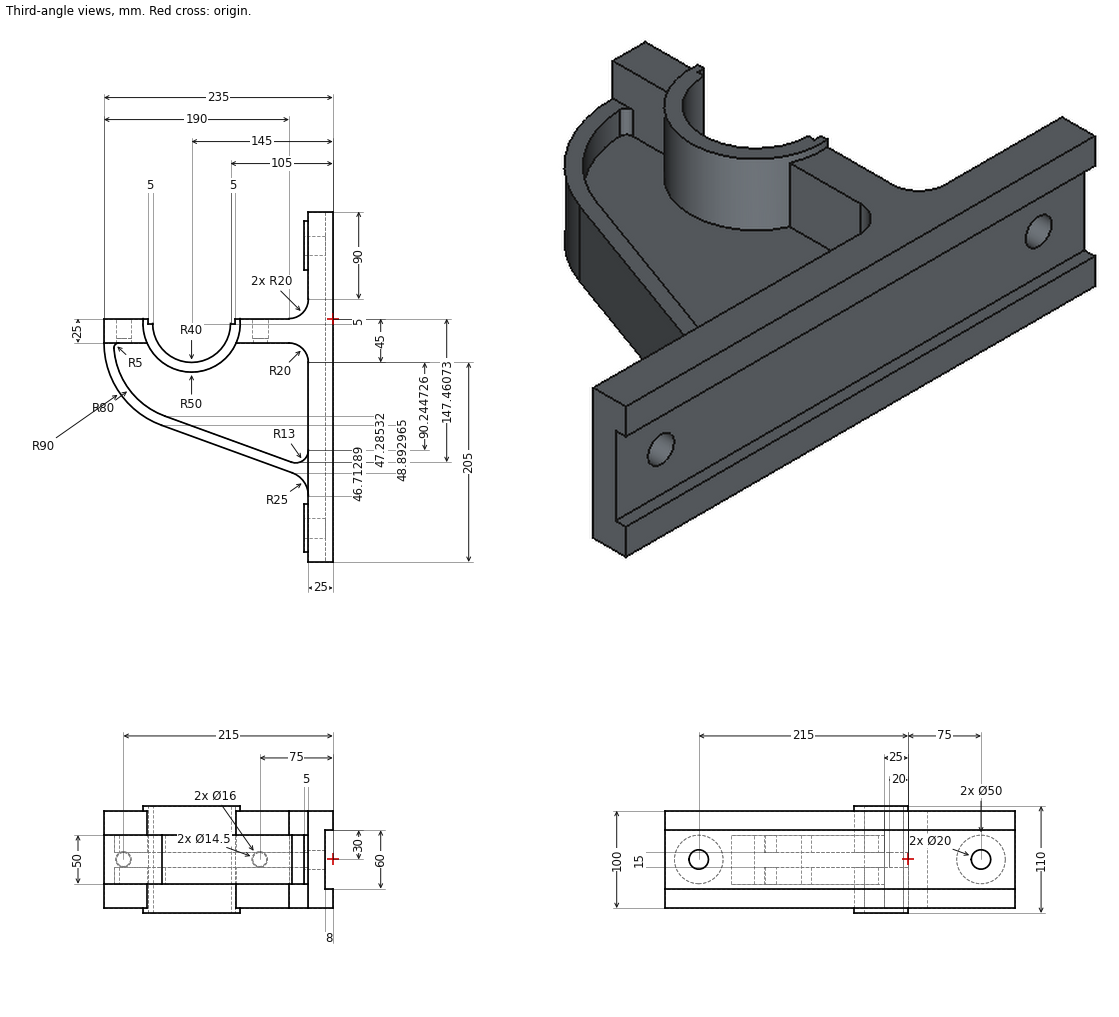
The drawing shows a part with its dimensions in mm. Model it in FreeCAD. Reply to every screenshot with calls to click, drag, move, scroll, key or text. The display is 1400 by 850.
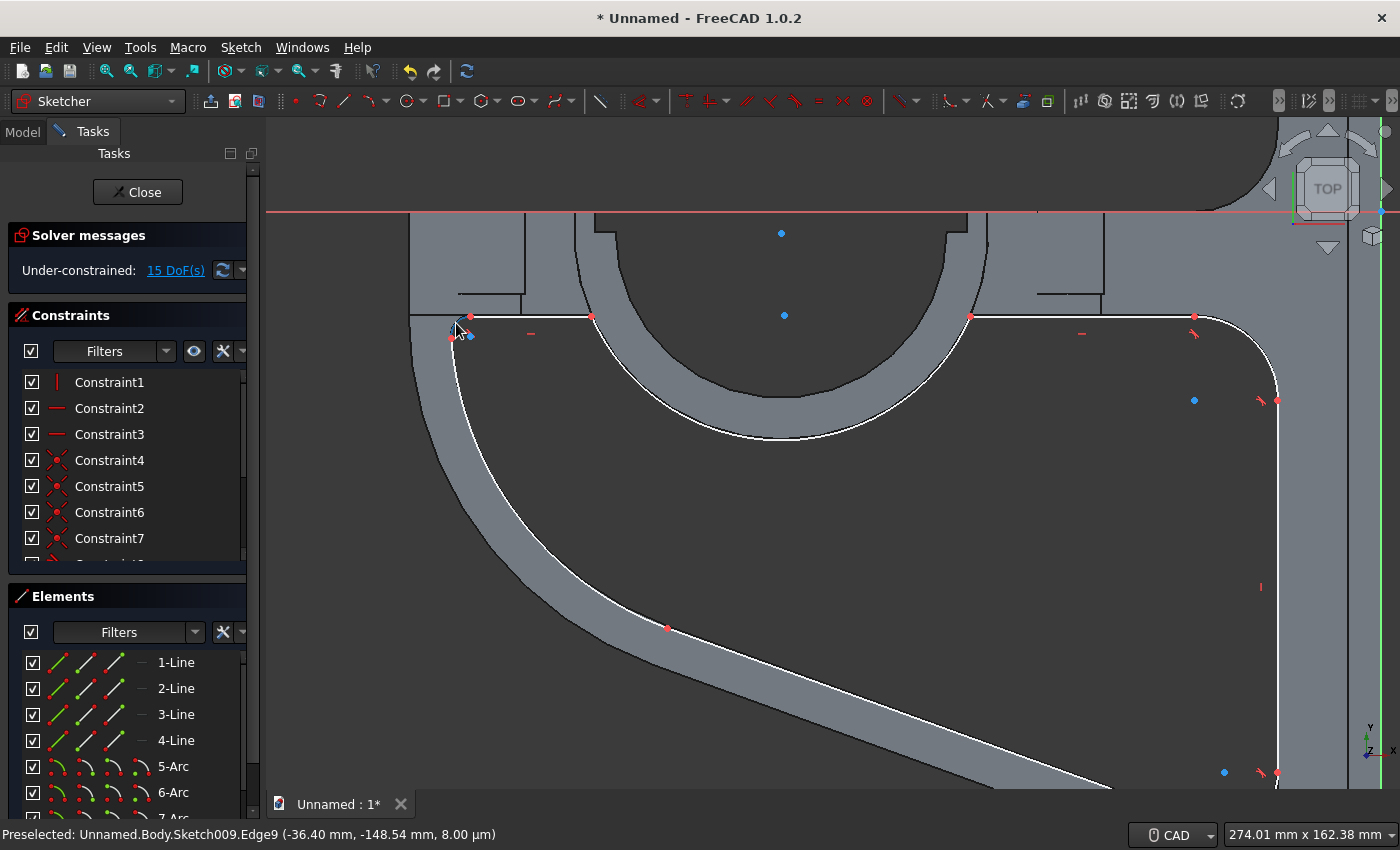
click(456, 323)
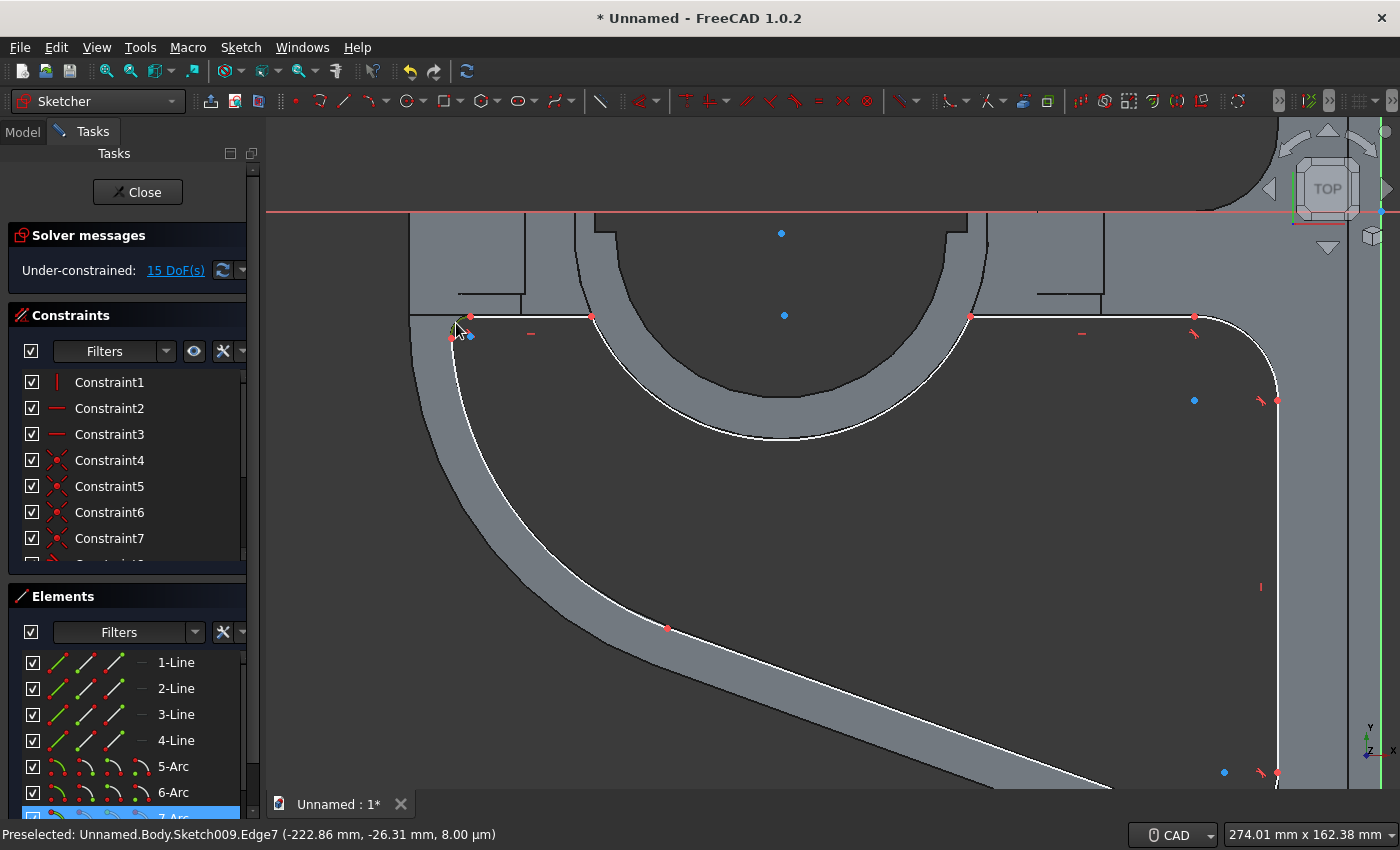
click(479, 450)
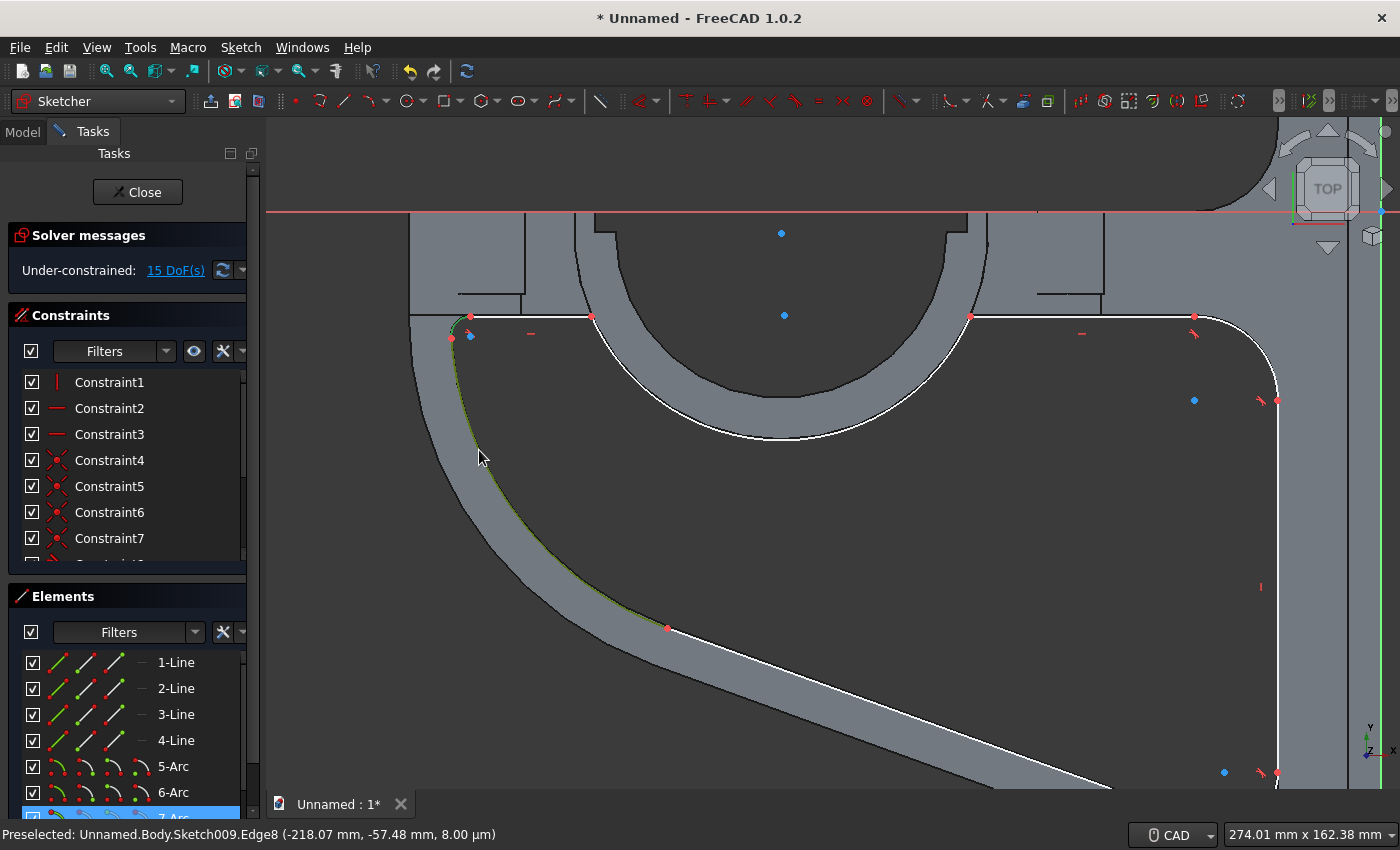
click(796, 102)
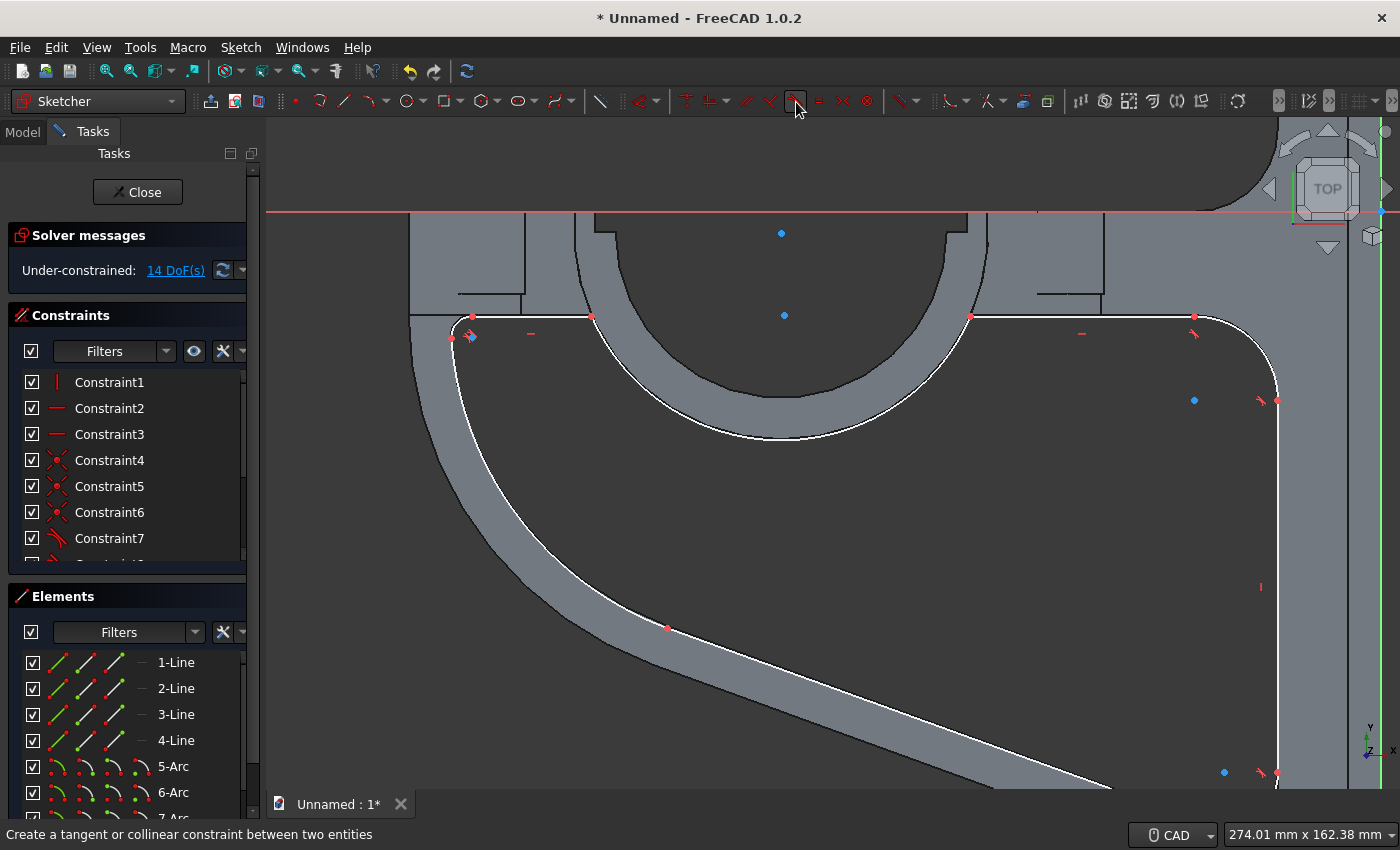
click(640, 102)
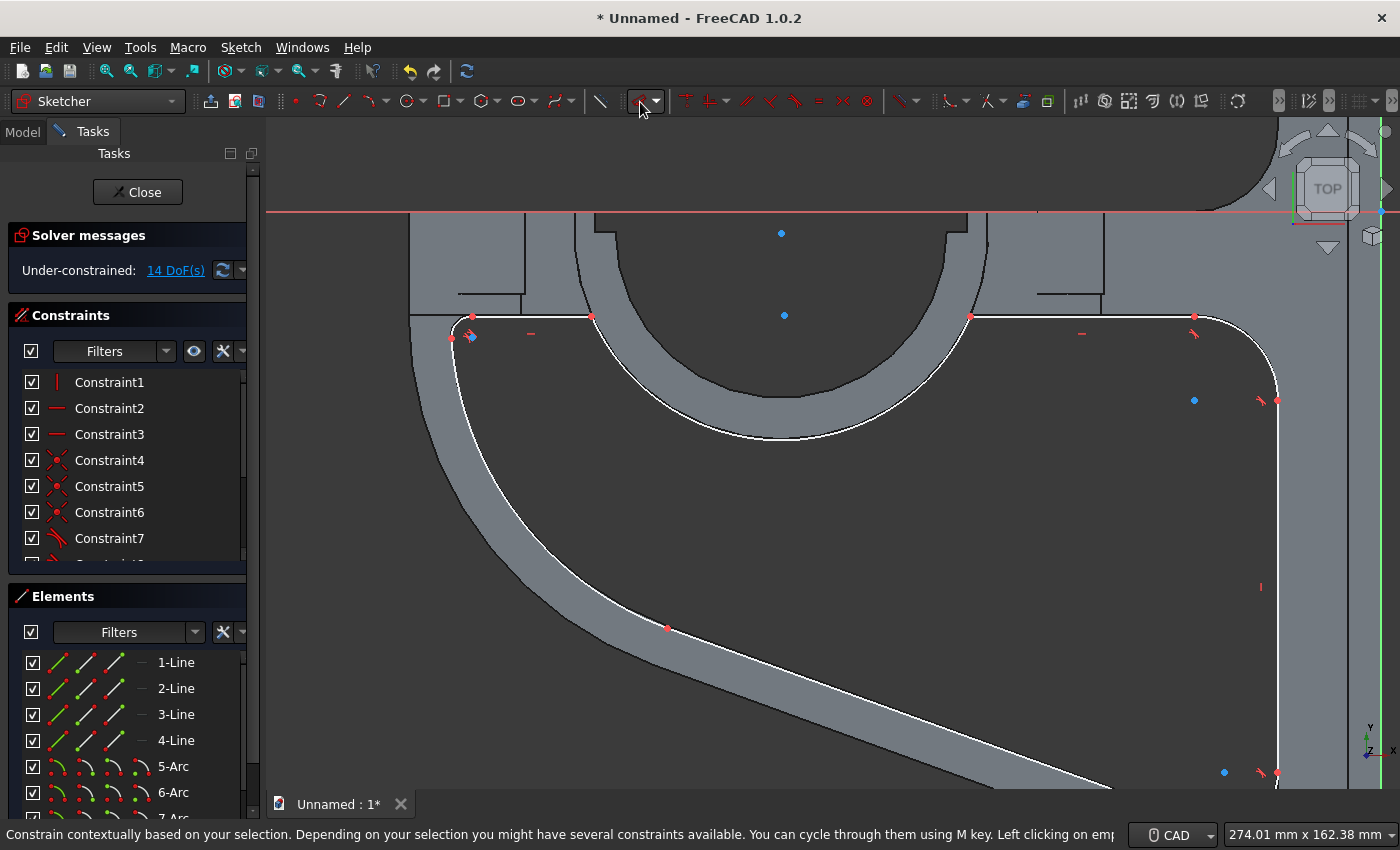
click(1232, 326)
click(1191, 285)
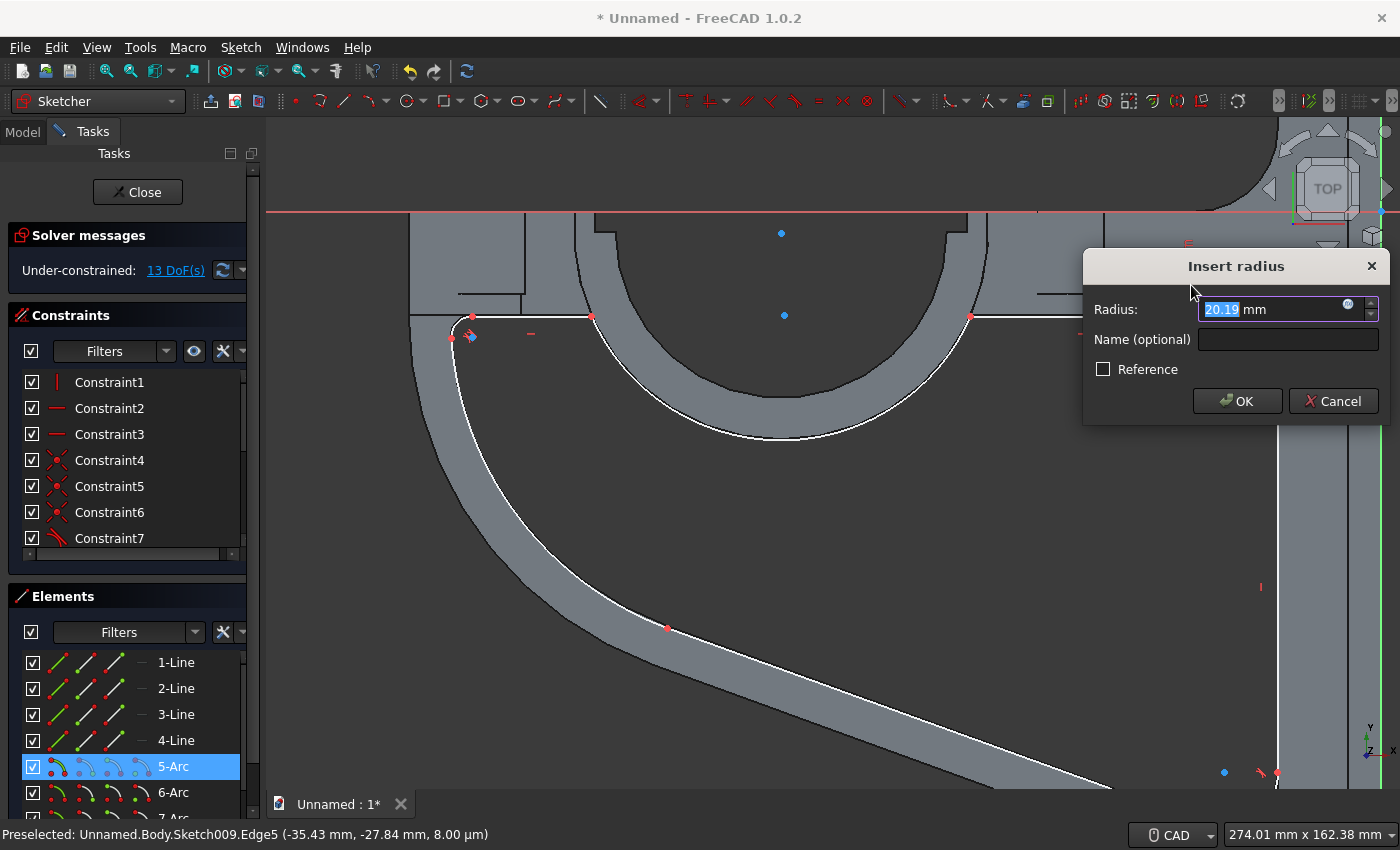
text(20)
key(Return)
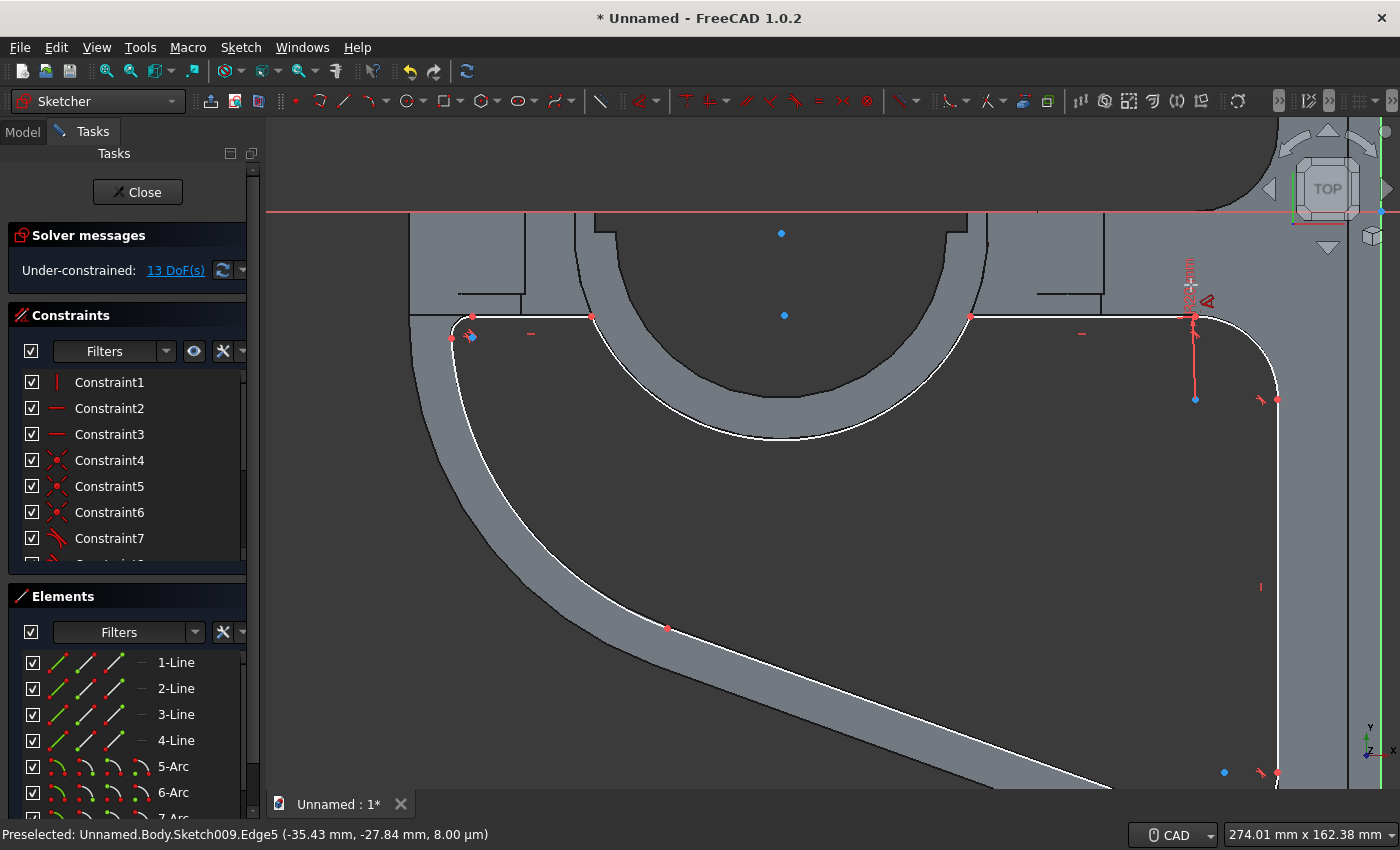
click(689, 419)
click(675, 448)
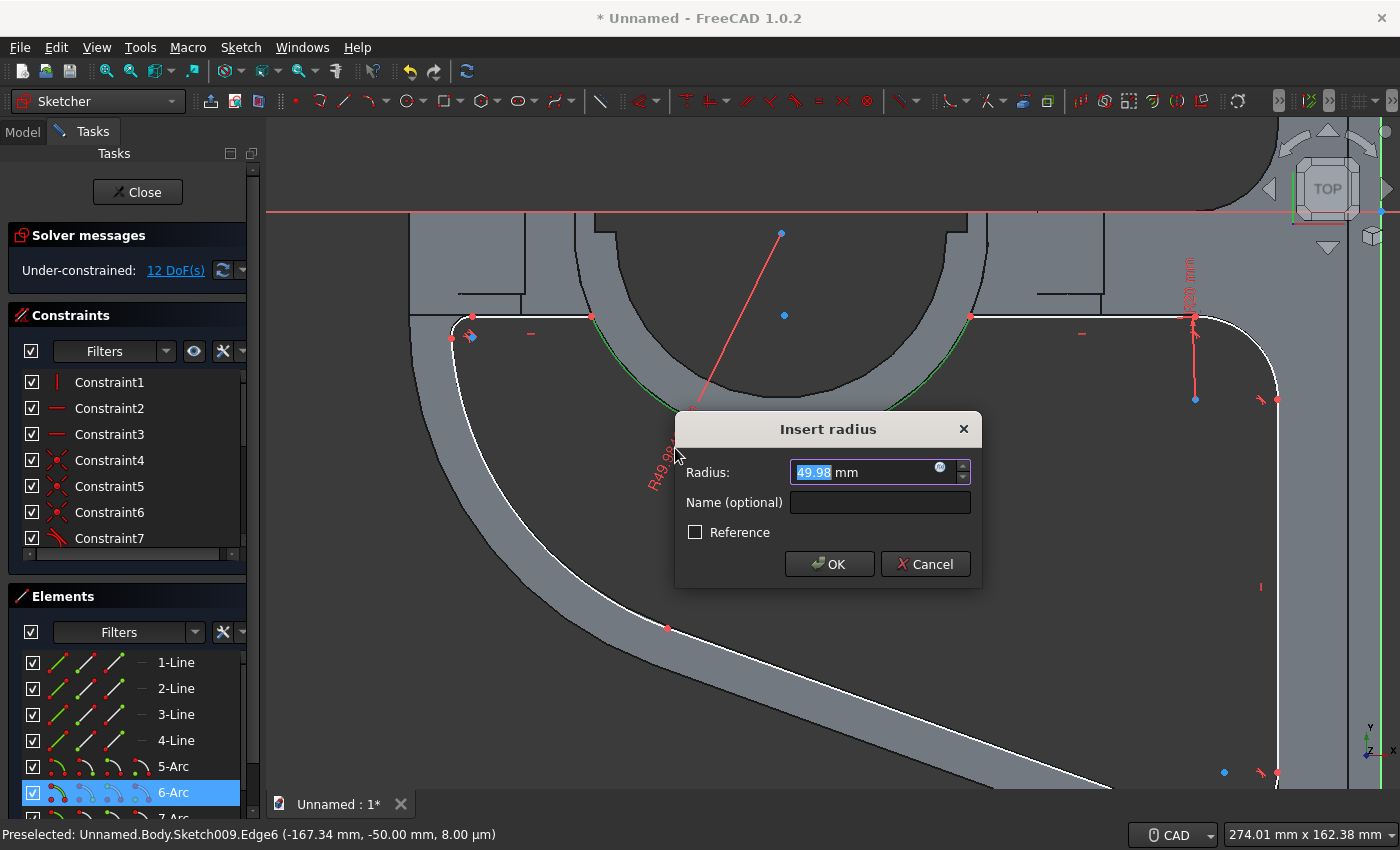
text(50)
key(Return)